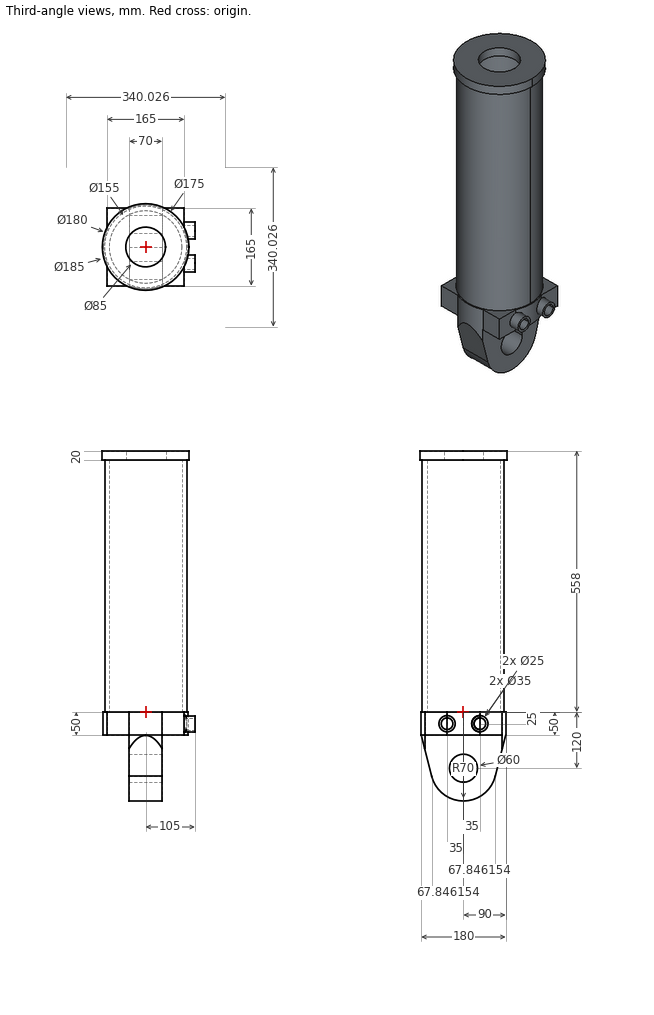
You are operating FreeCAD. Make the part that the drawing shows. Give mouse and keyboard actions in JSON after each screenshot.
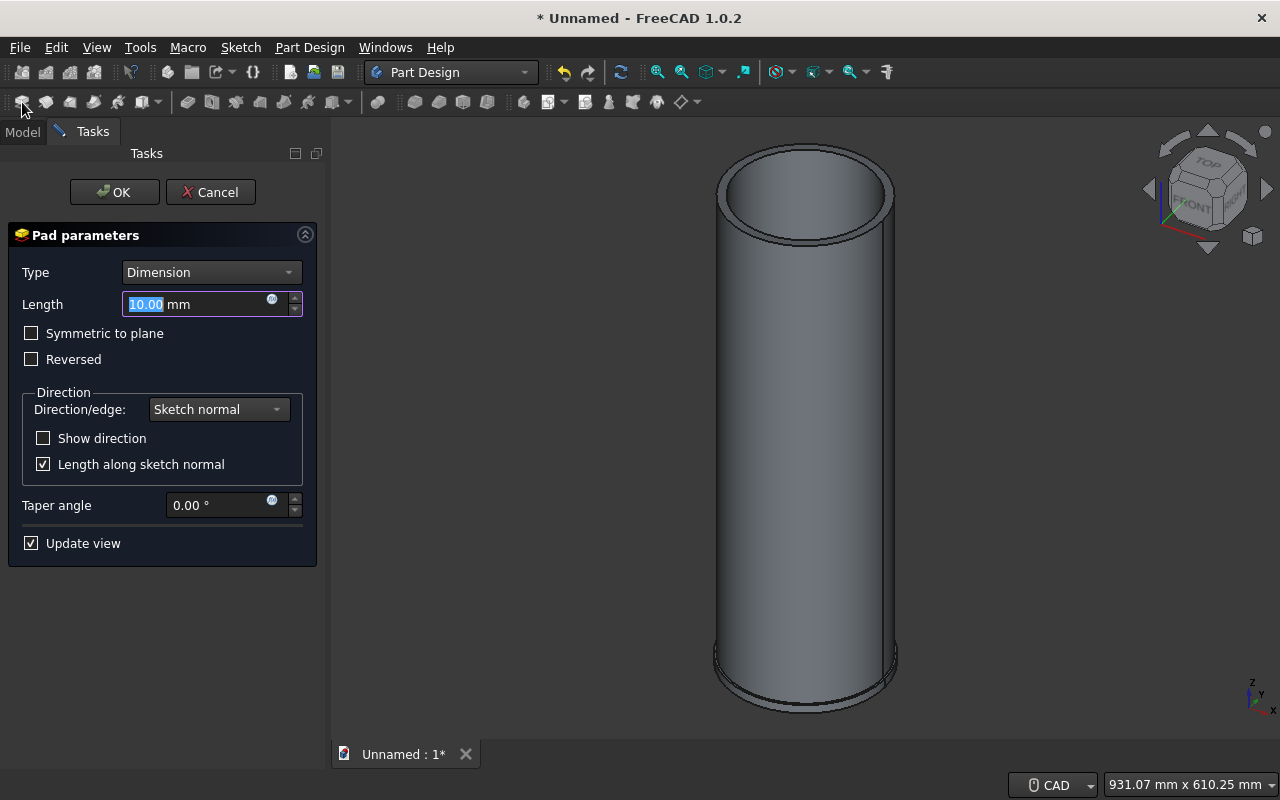
{"action": "type", "text": "50"}
{"action": "key", "text": "Tab"}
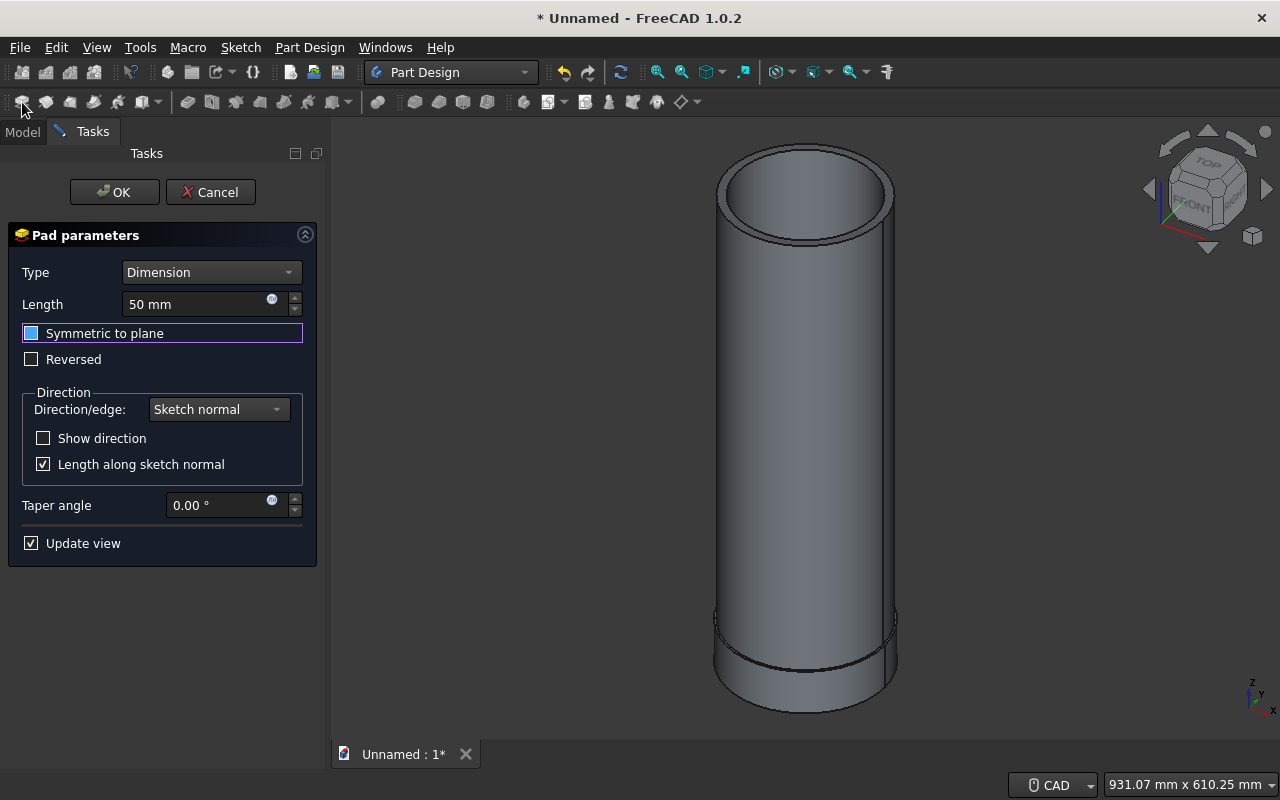
{"action": "left_click", "coordinate": [30, 359]}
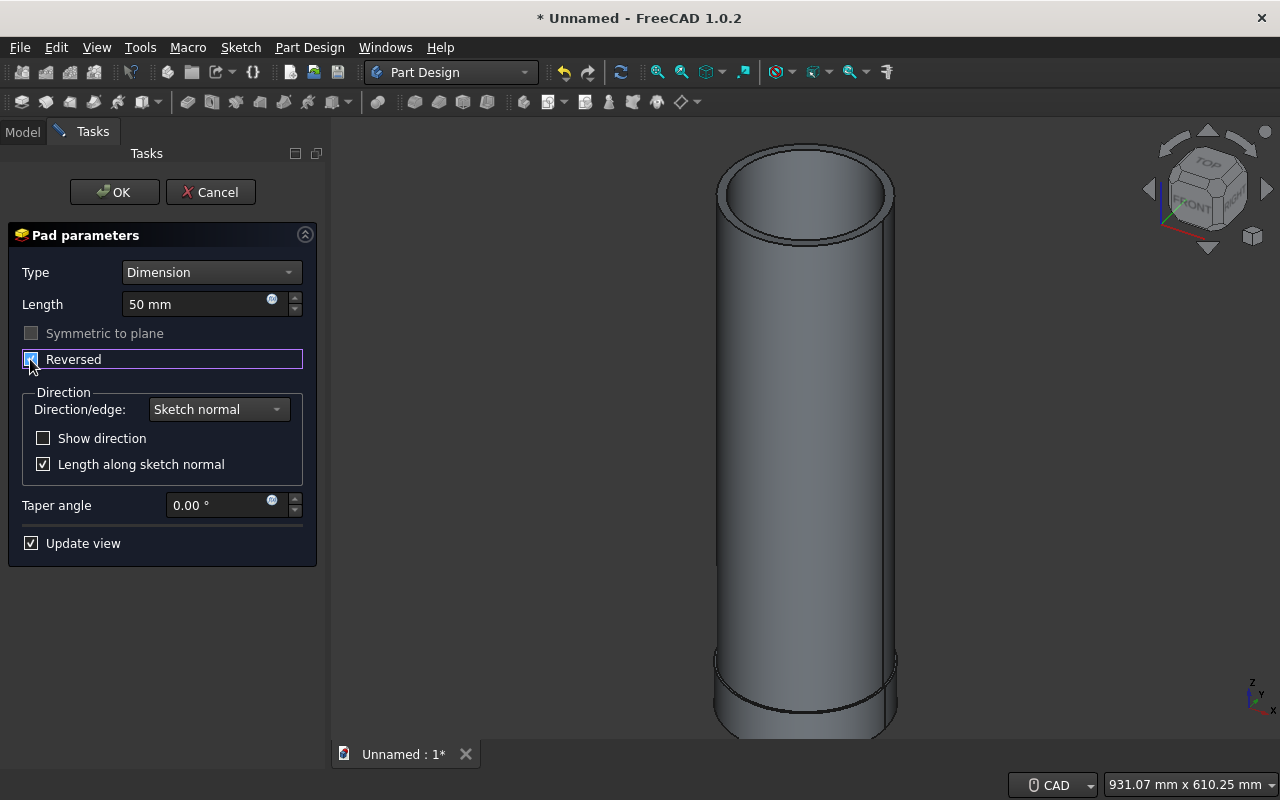
{"action": "left_click", "coordinate": [115, 192]}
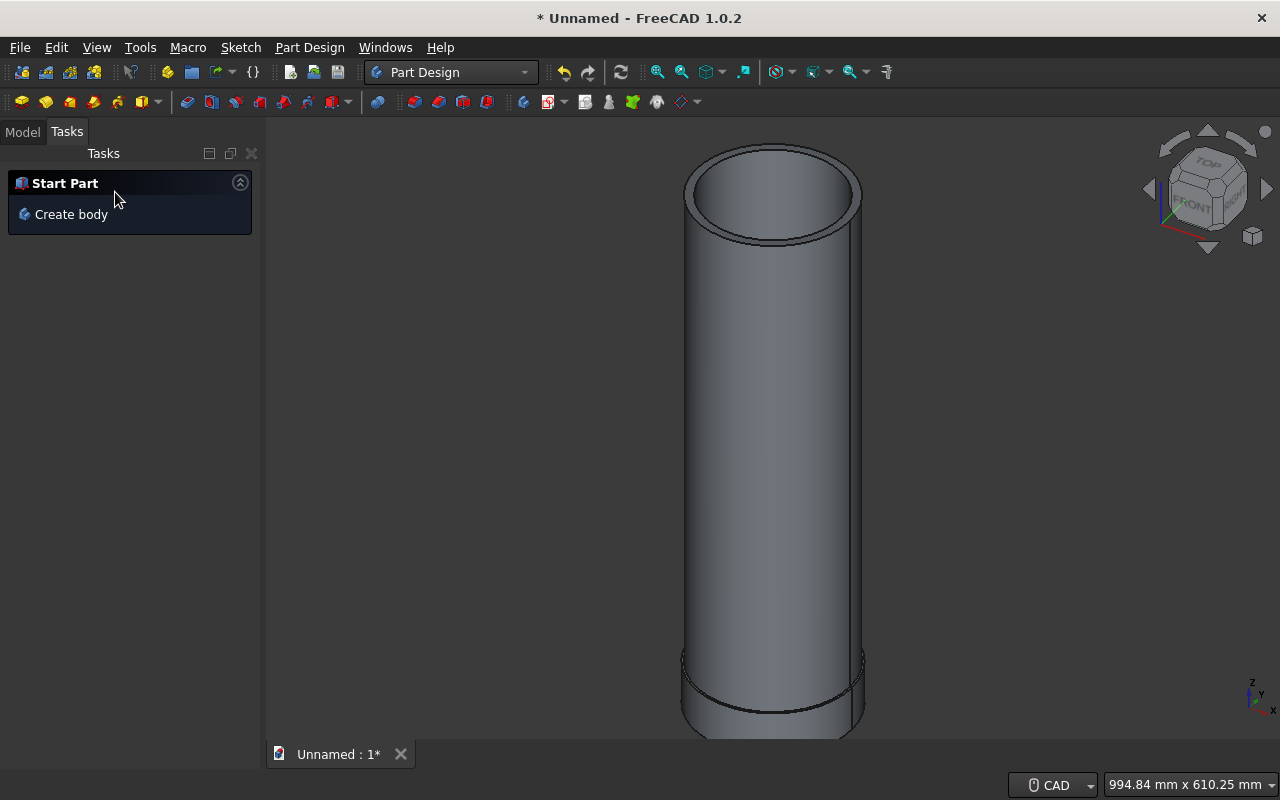
{"action": "left_click", "coordinate": [658, 72]}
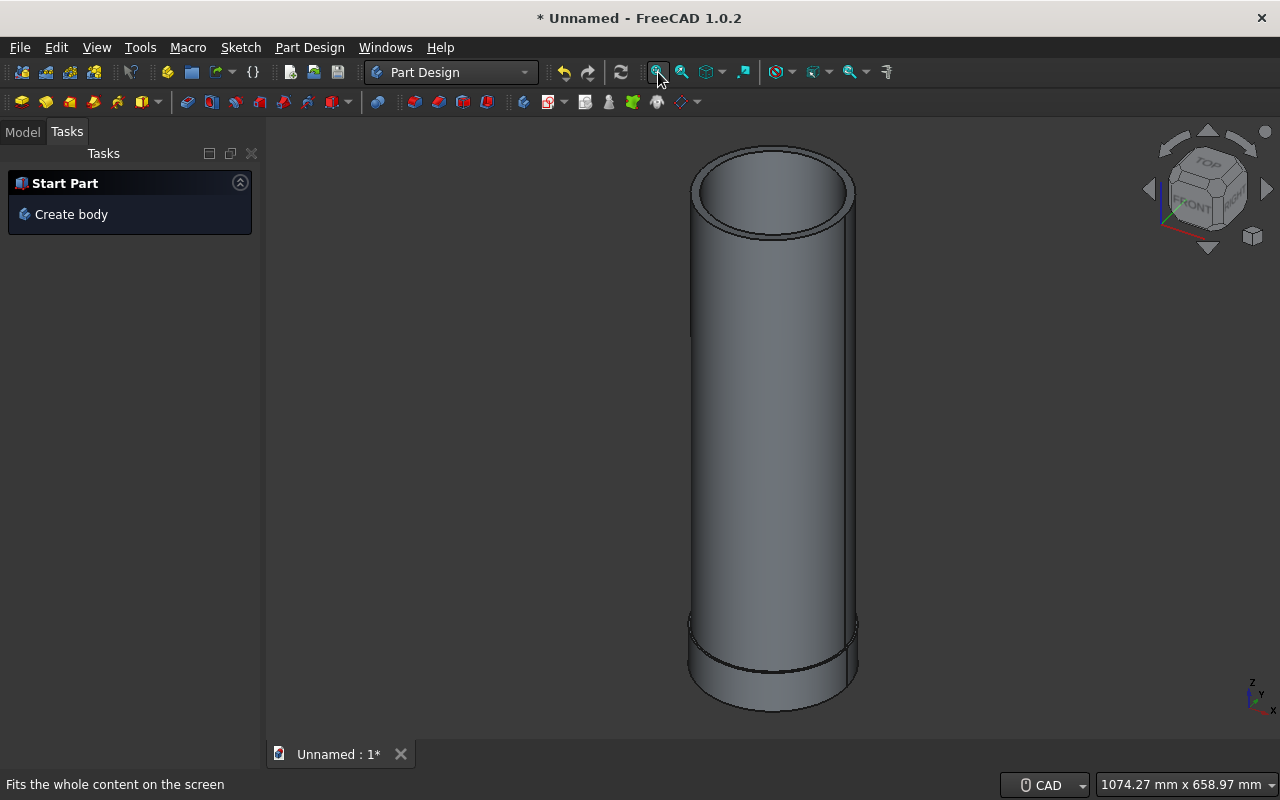
{"action": "left_click", "coordinate": [548, 102]}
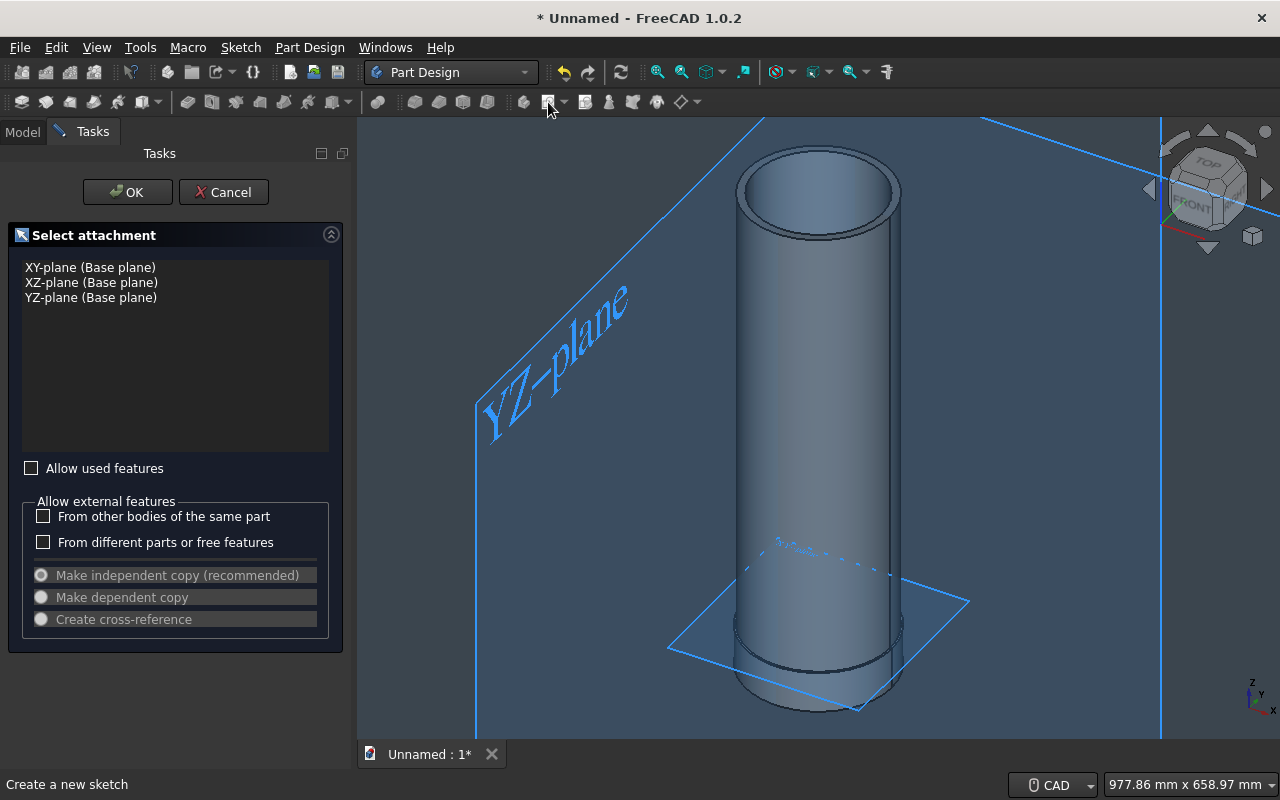
{"action": "left_click", "coordinate": [82, 298]}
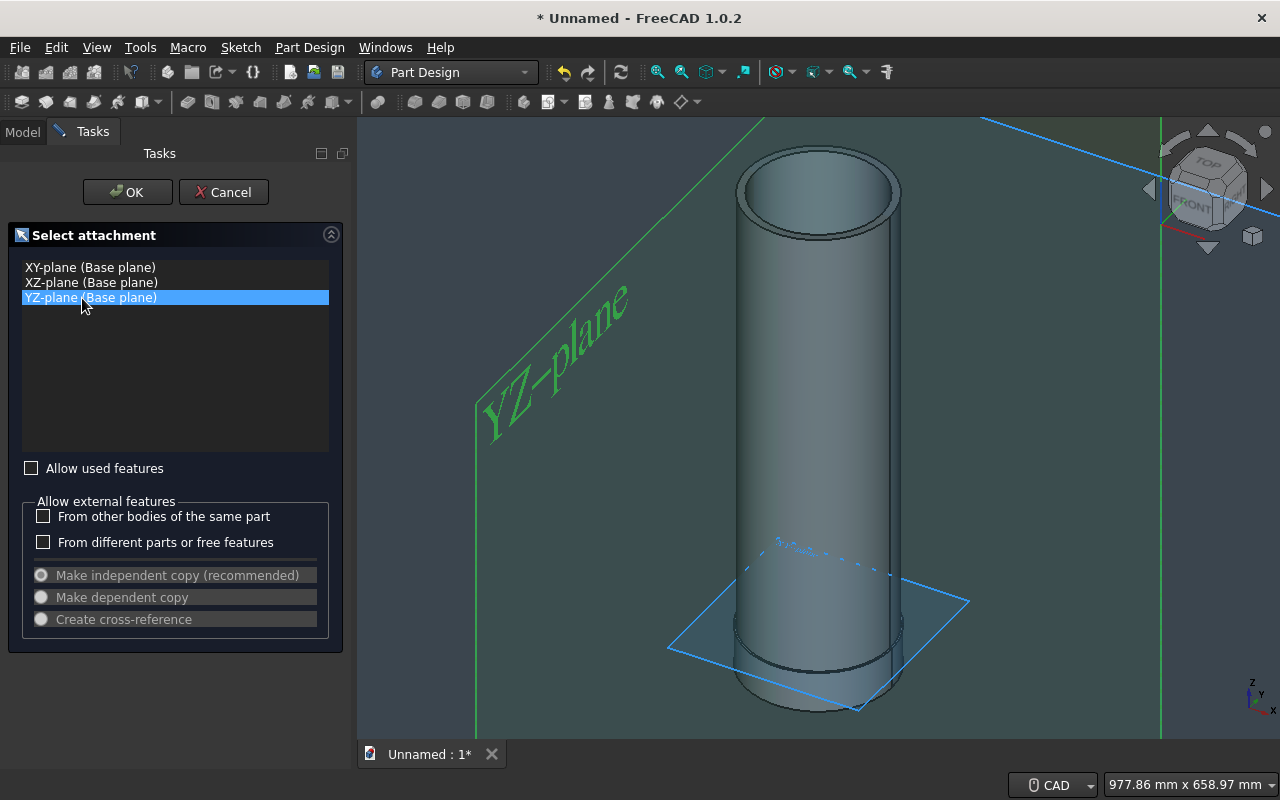
{"action": "left_click", "coordinate": [128, 192]}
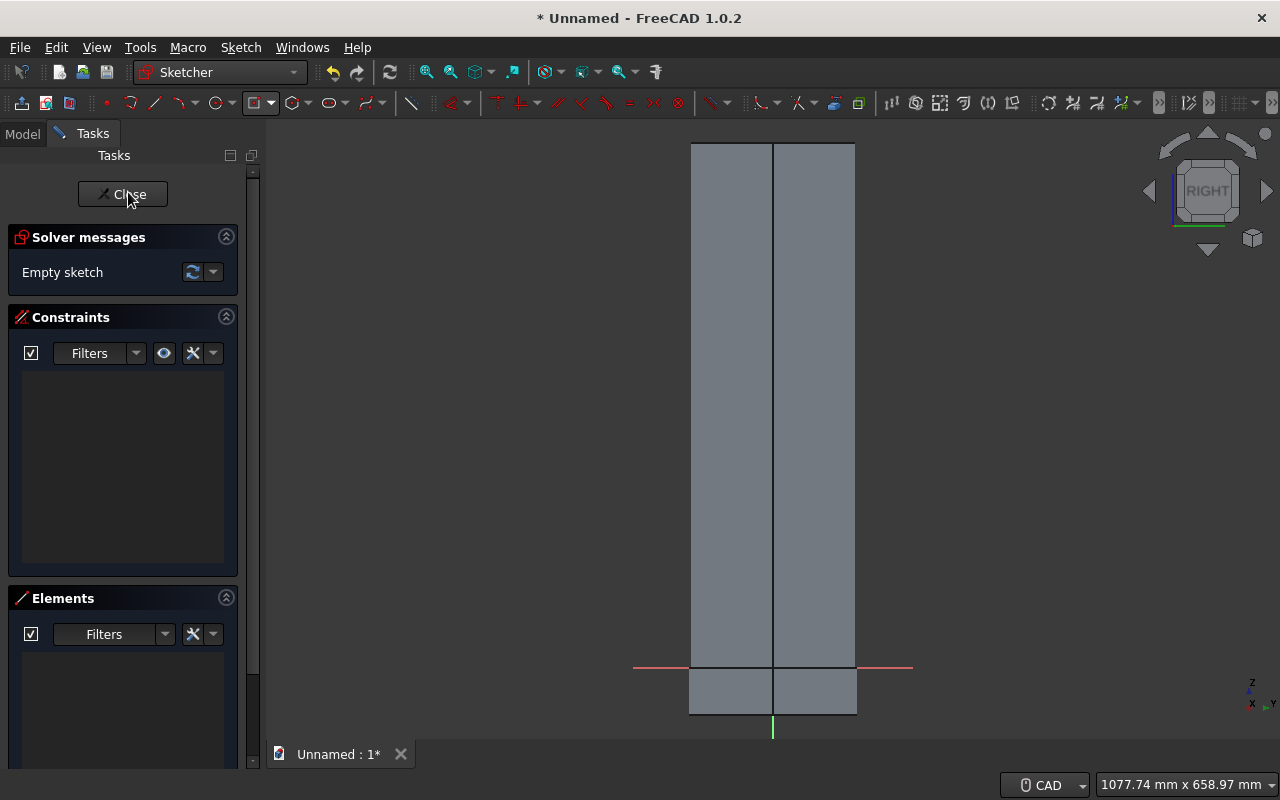
{"action": "left_click", "coordinate": [70, 104]}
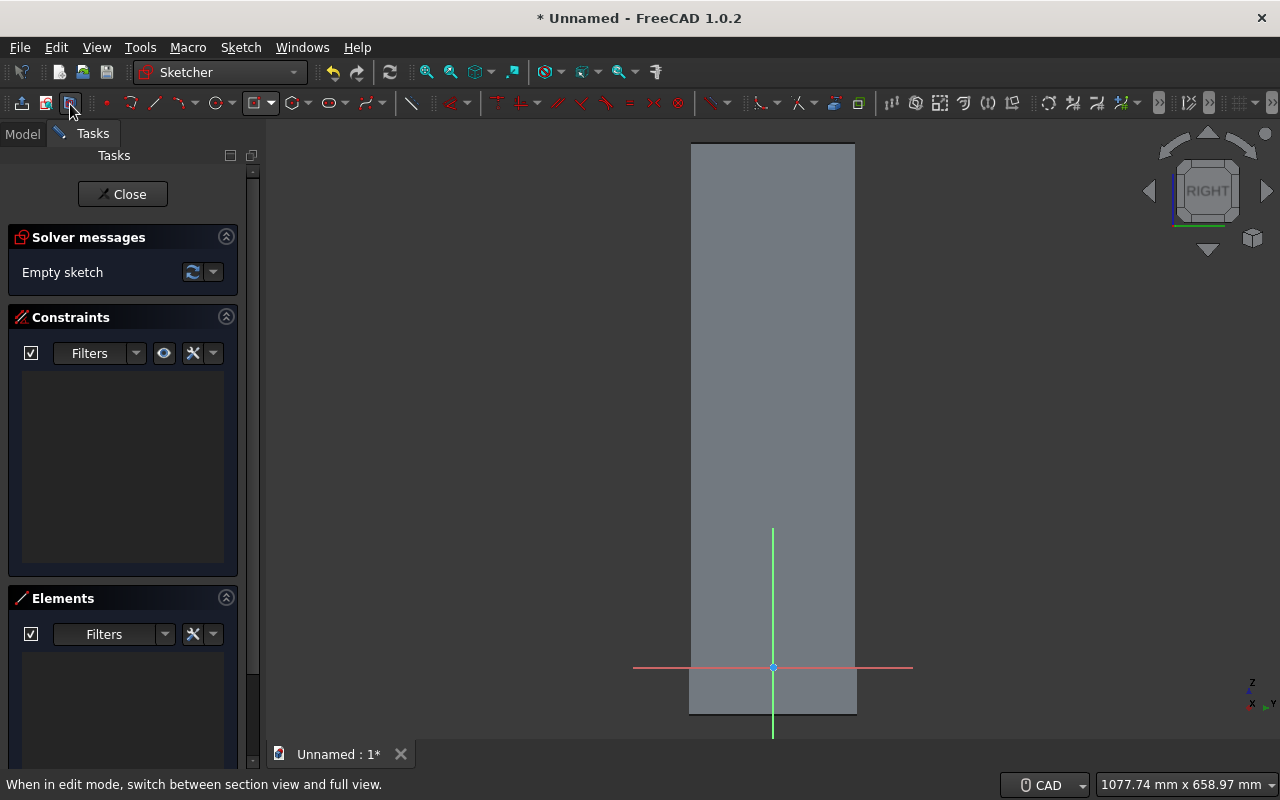
{"action": "scroll", "coordinate": [704, 429], "scroll_direction": "down", "scroll_amount": 5}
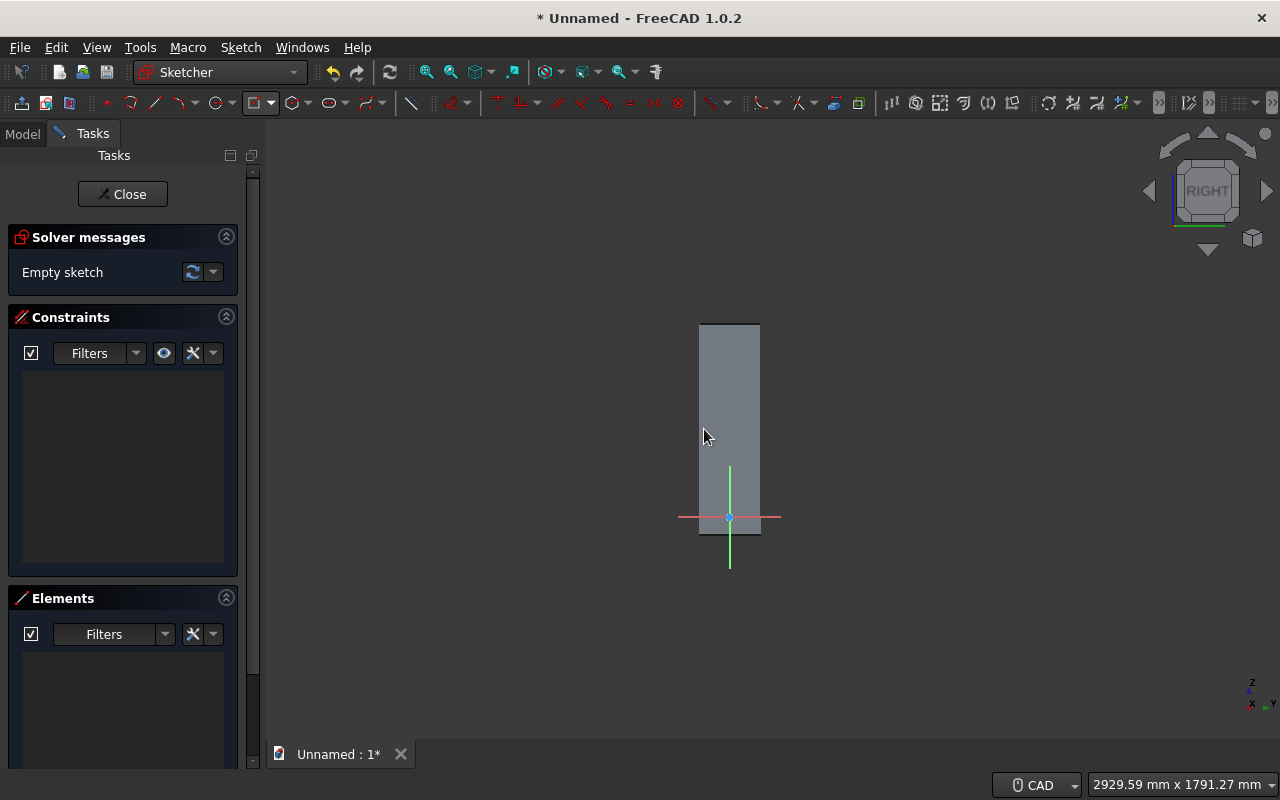
{"action": "scroll", "coordinate": [735, 574], "scroll_direction": "up", "scroll_amount": 9}